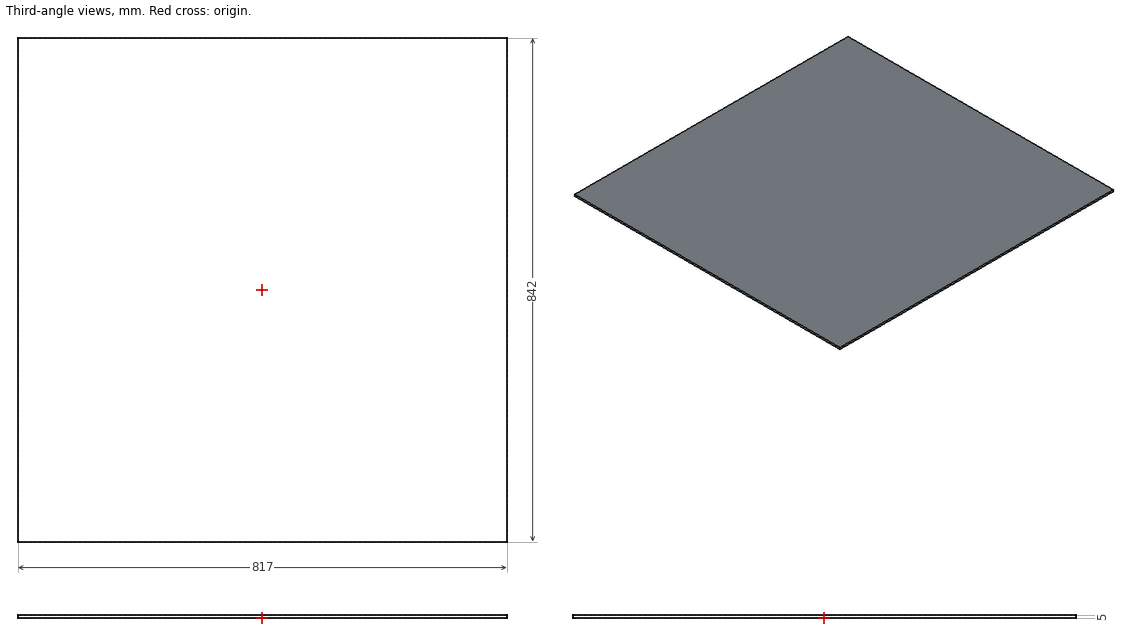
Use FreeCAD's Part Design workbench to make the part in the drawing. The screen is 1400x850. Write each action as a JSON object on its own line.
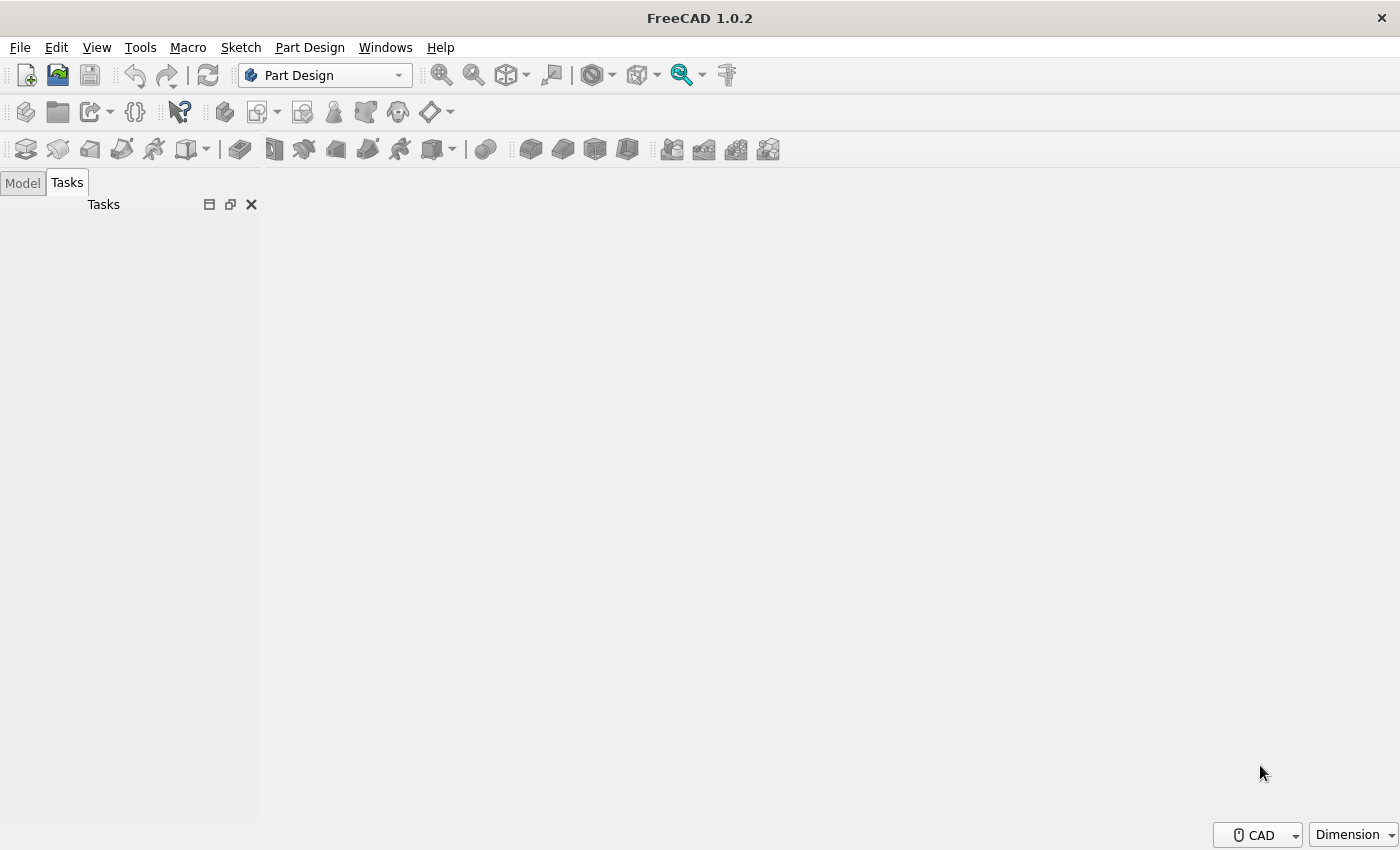
{"action": "left_click", "coordinate": [26, 76]}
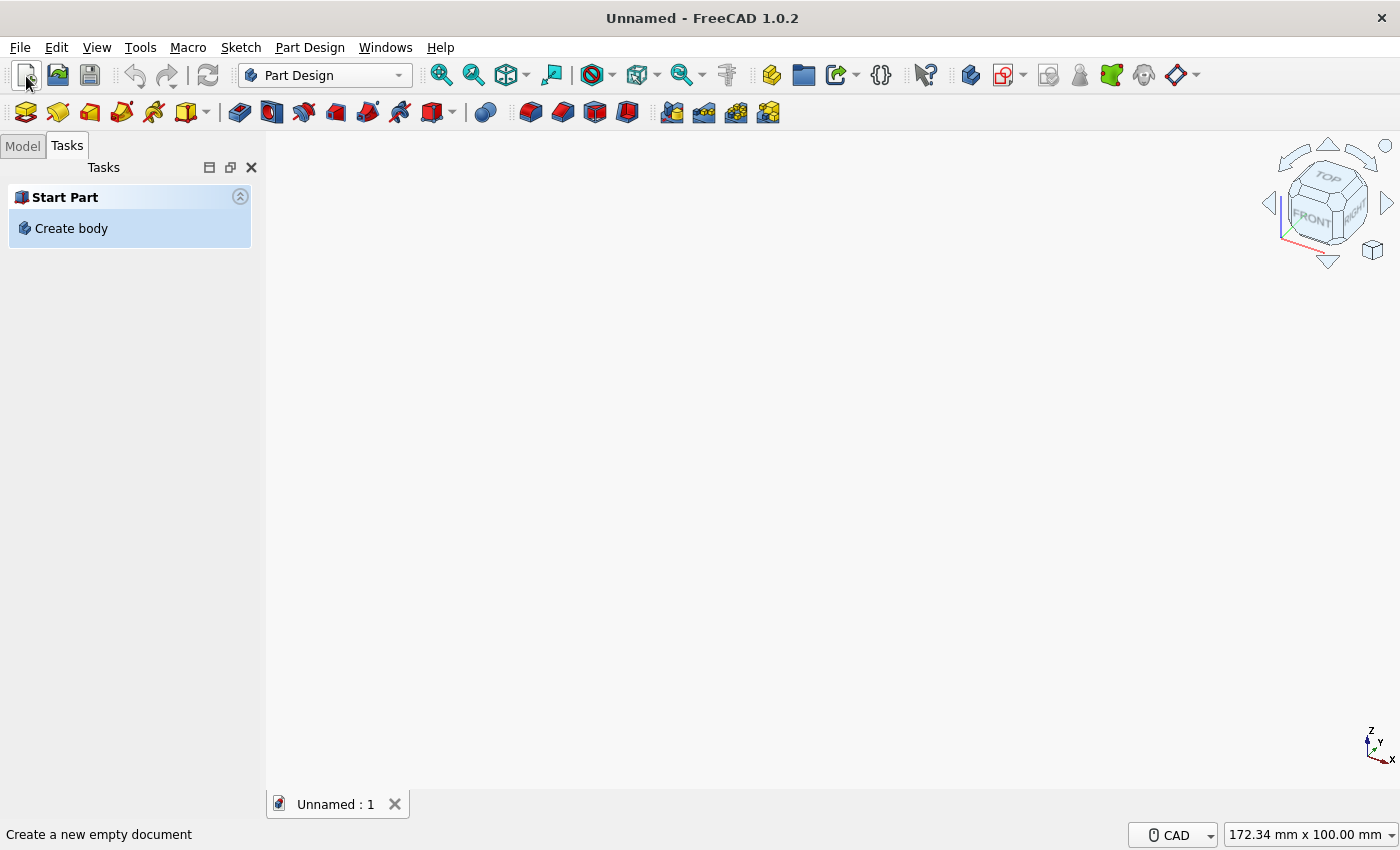
{"action": "left_click", "coordinate": [1004, 76]}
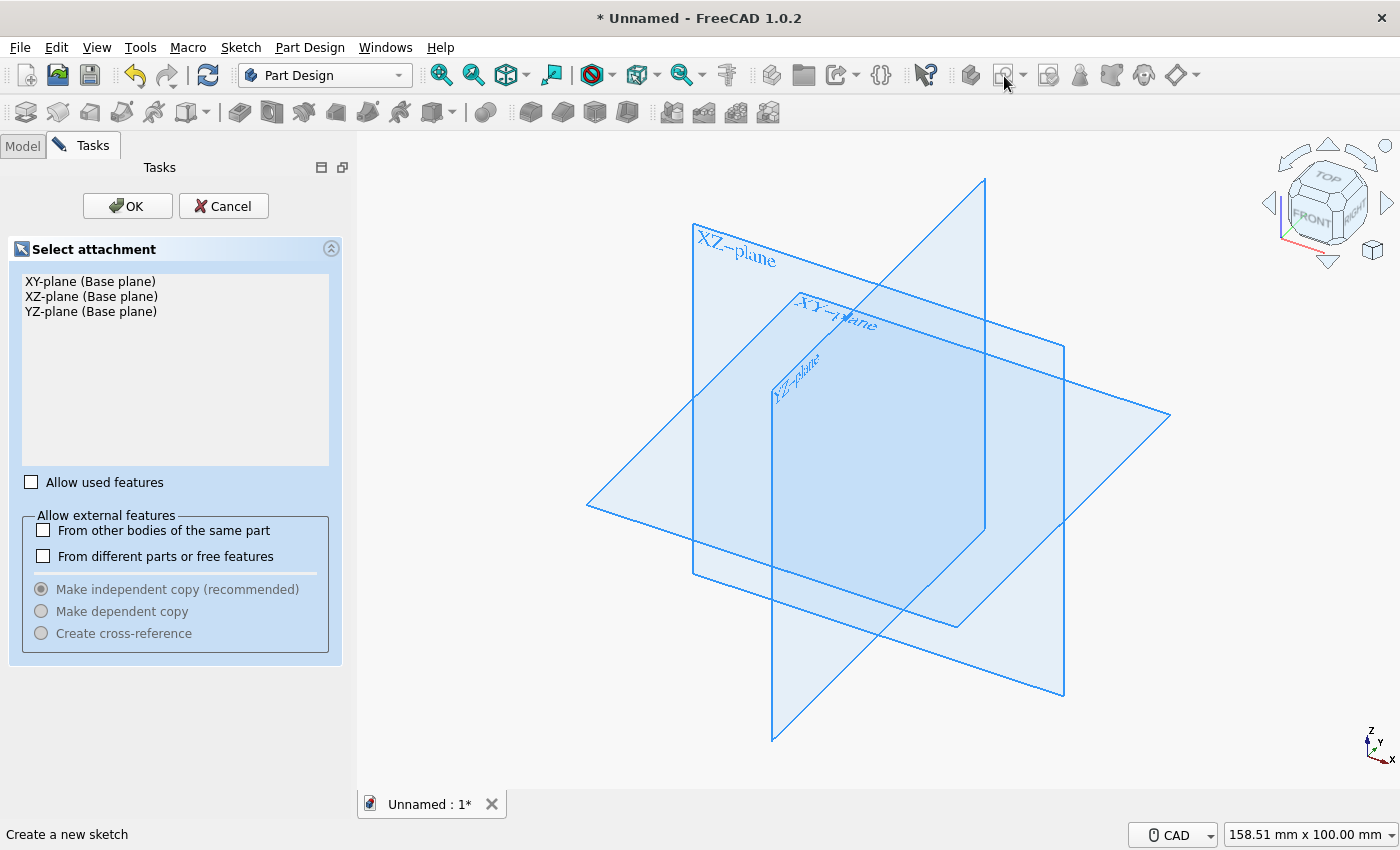
{"action": "left_click", "coordinate": [82, 282]}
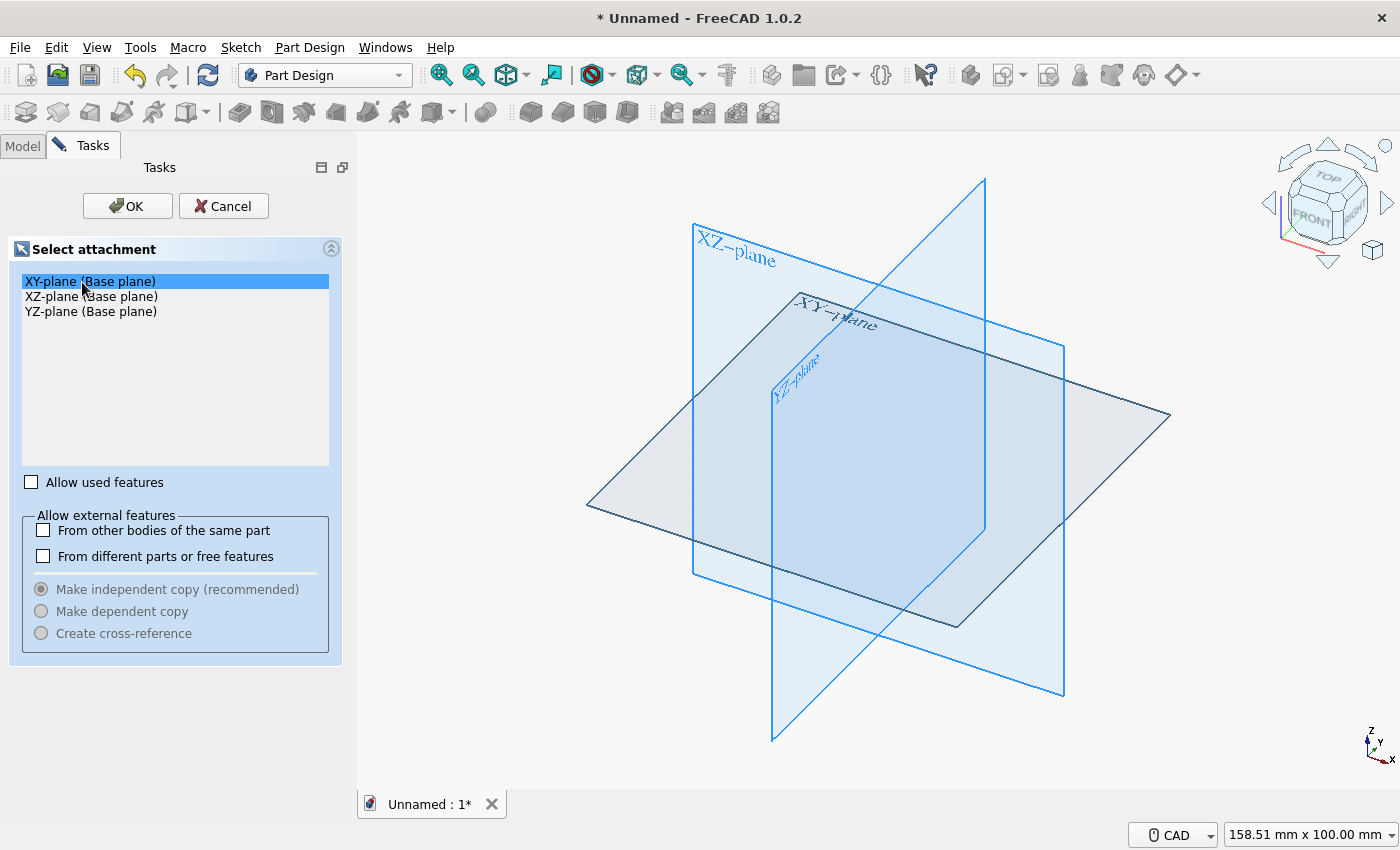
{"action": "left_click", "coordinate": [128, 206]}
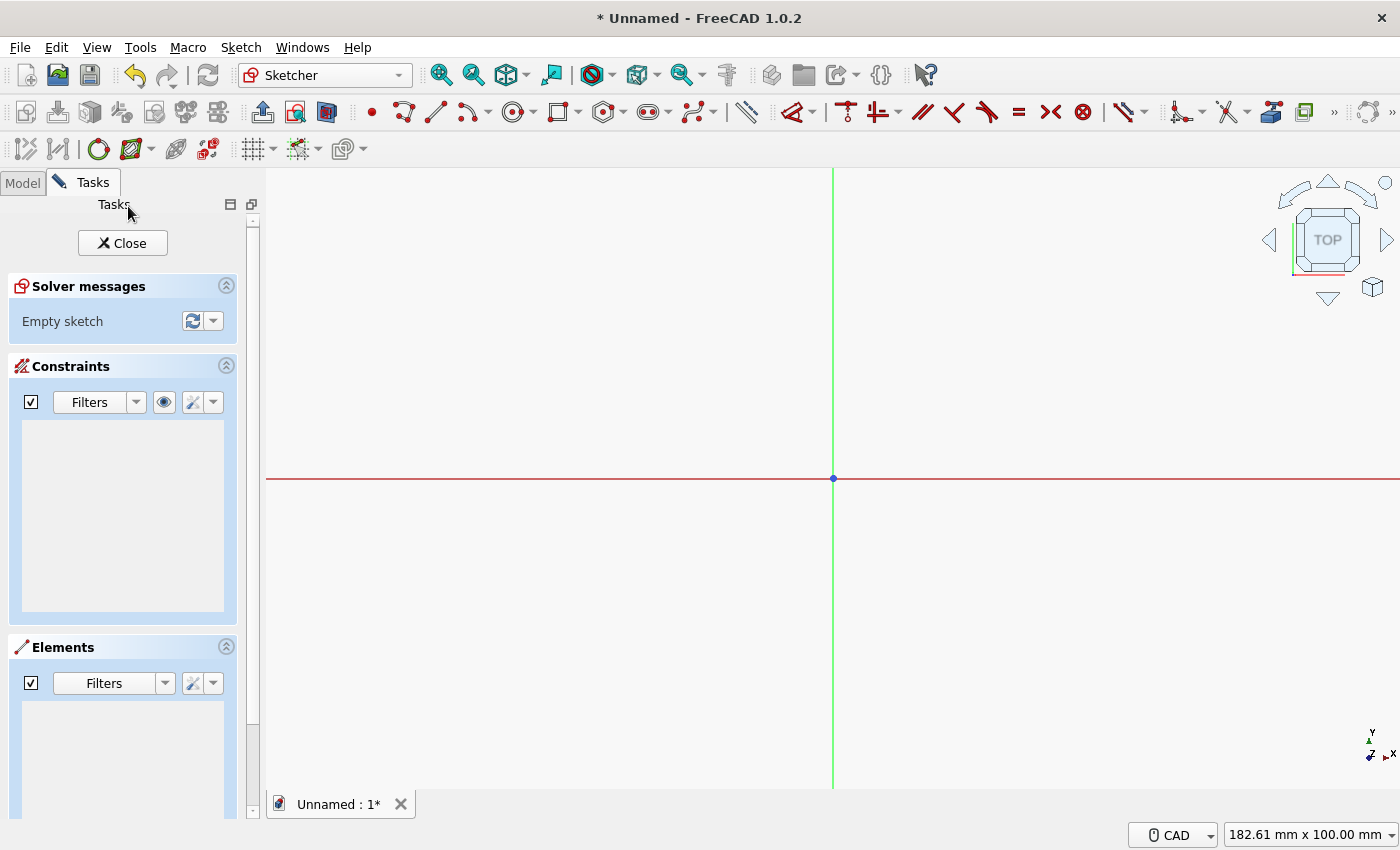
{"action": "scroll", "coordinate": [759, 478], "scroll_direction": "down", "scroll_amount": 13}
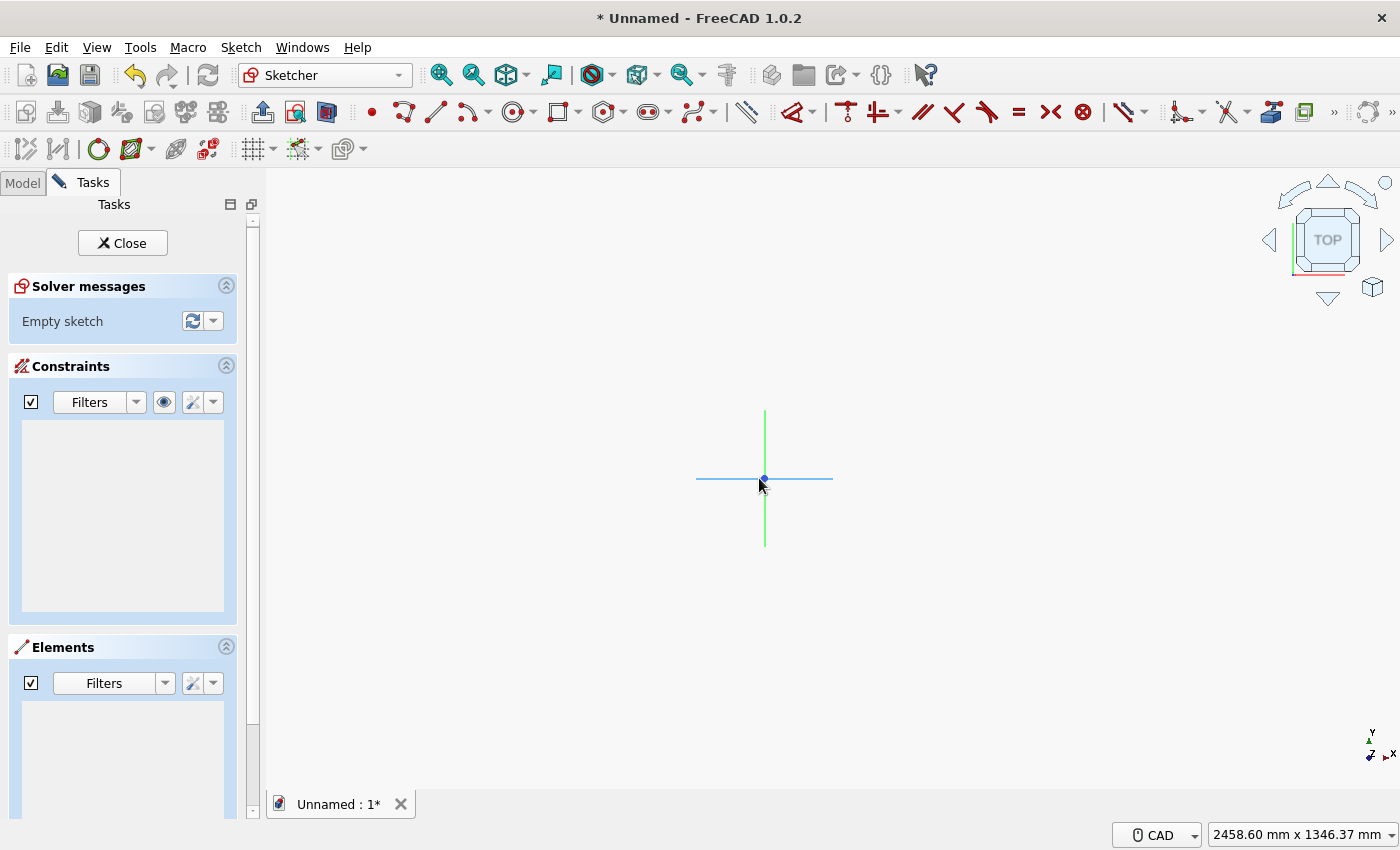
{"action": "key", "text": "g v"}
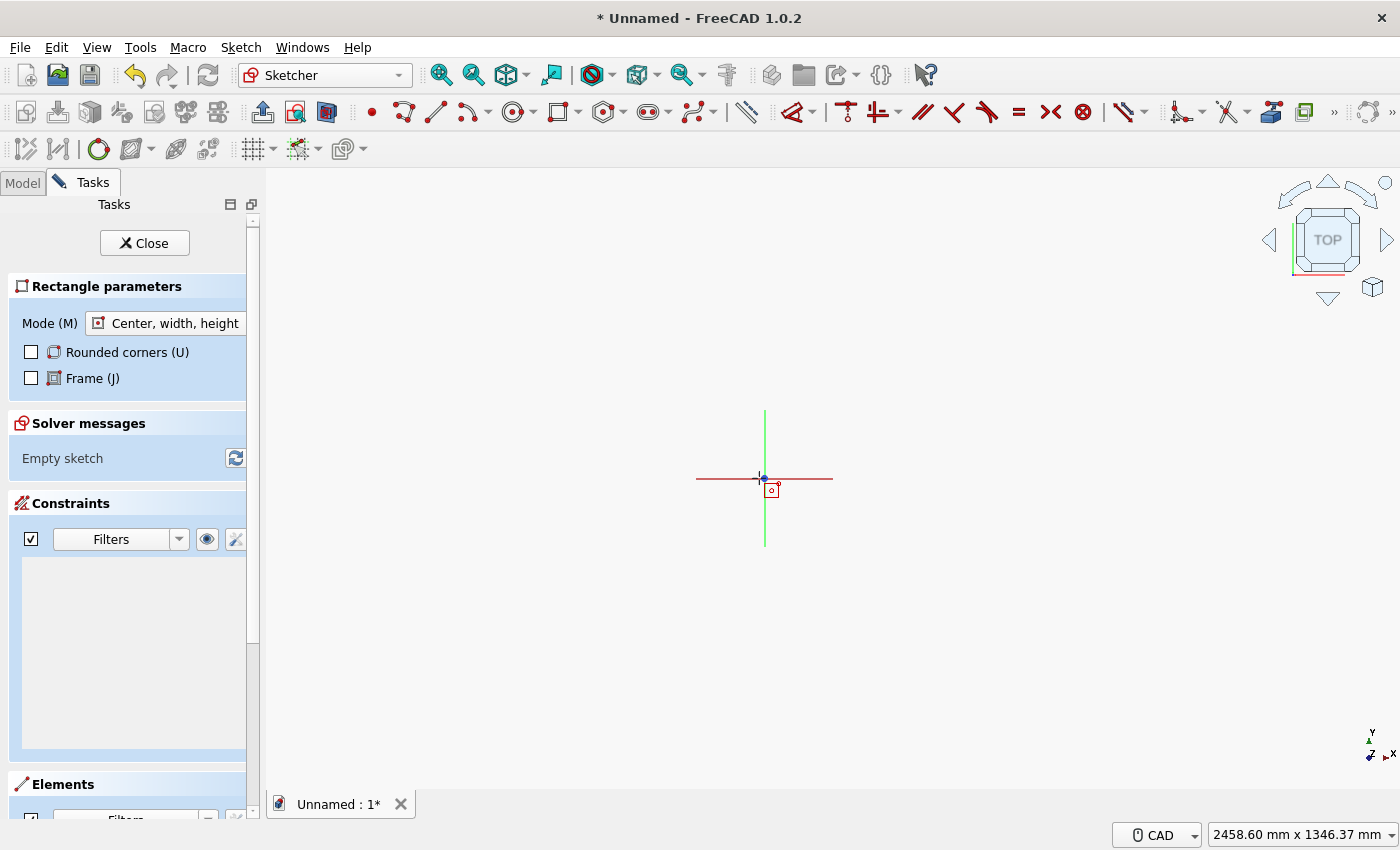
{"action": "left_click", "coordinate": [765, 478]}
{"action": "mouse_move", "coordinate": [953, 284]}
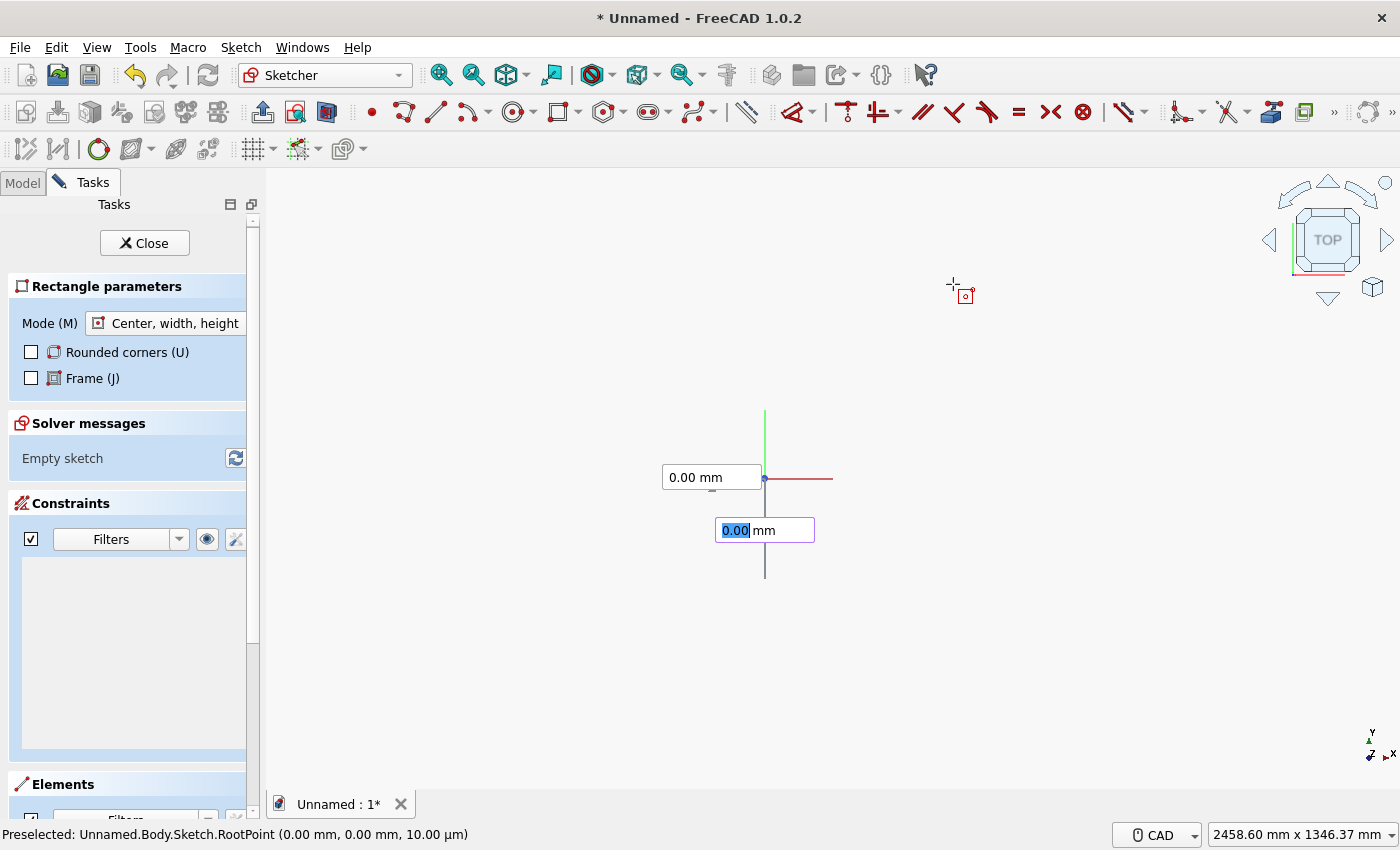
{"action": "type", "text": "817"}
{"action": "key", "text": "Tab"}
{"action": "type", "text": "842"}
{"action": "key", "text": "Return"}
{"action": "key", "text": "Escape"}